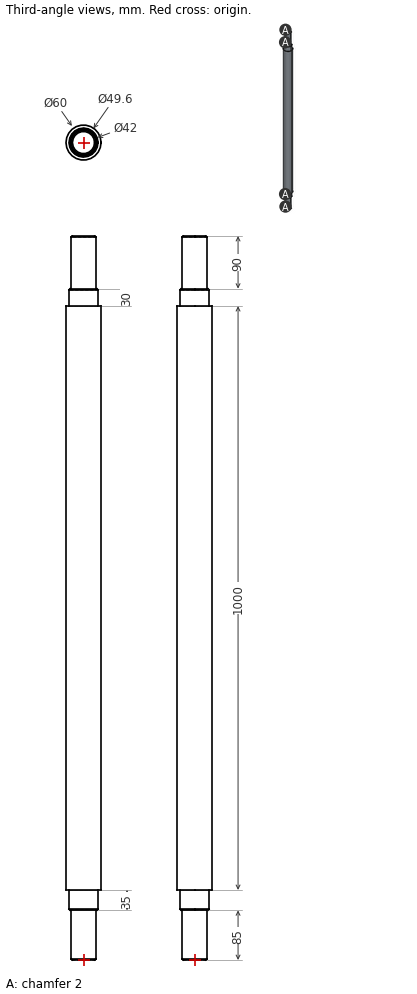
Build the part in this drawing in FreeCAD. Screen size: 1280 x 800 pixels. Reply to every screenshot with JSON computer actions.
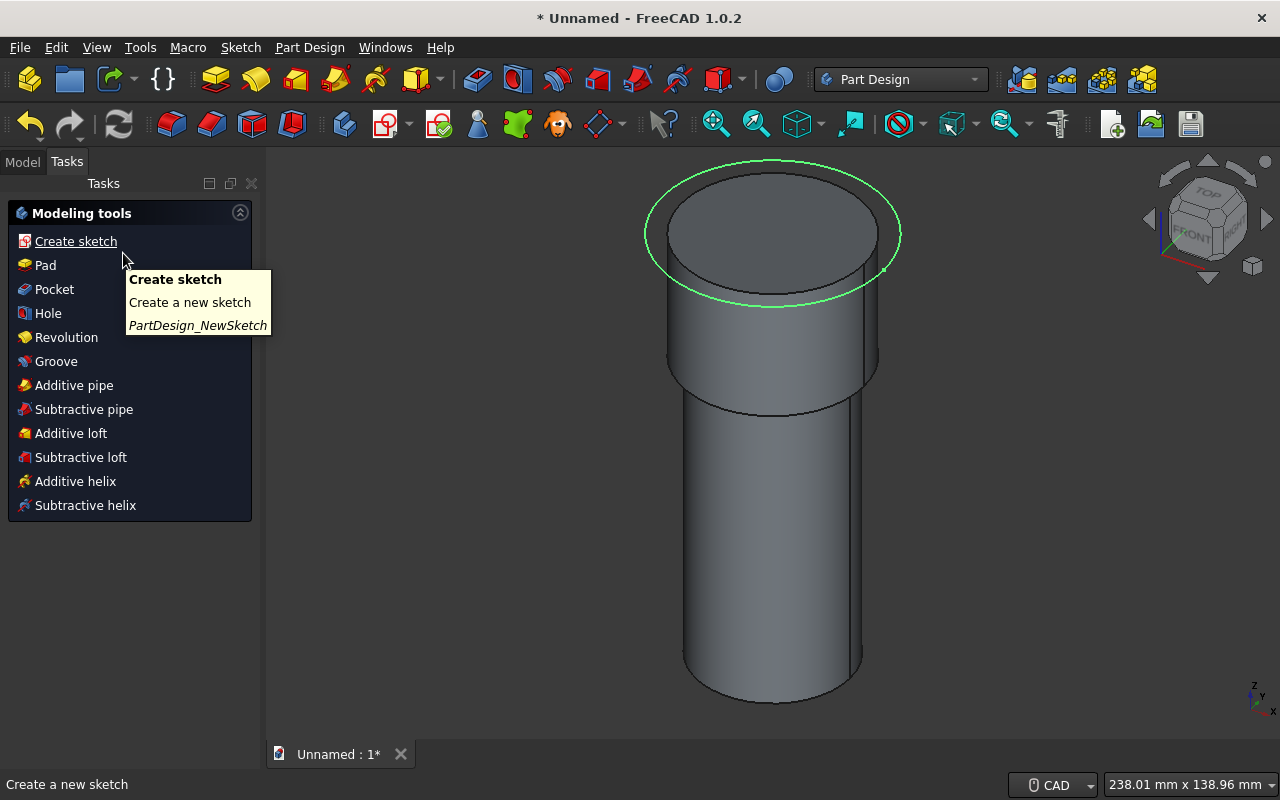
{"action": "left_click", "coordinate": [216, 80]}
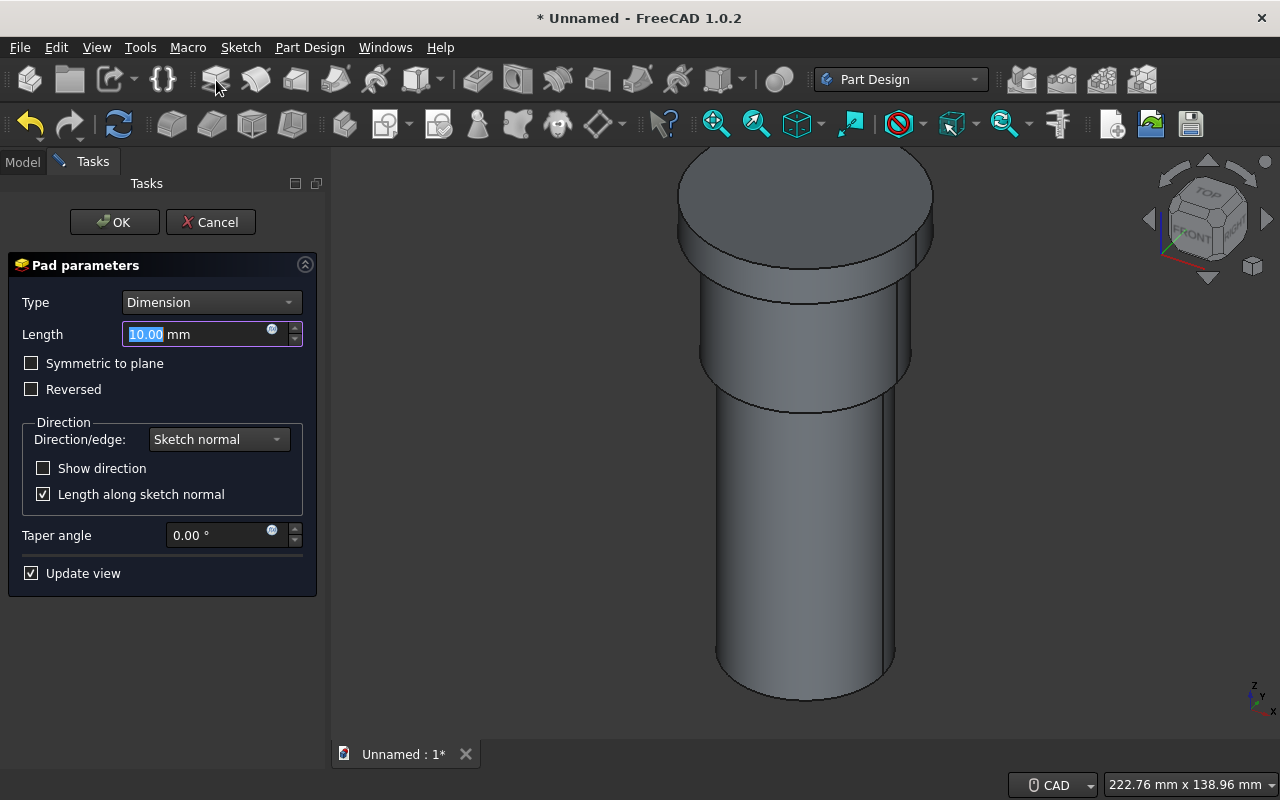
{"action": "type", "text": "1000"}
{"action": "key", "text": "Tab"}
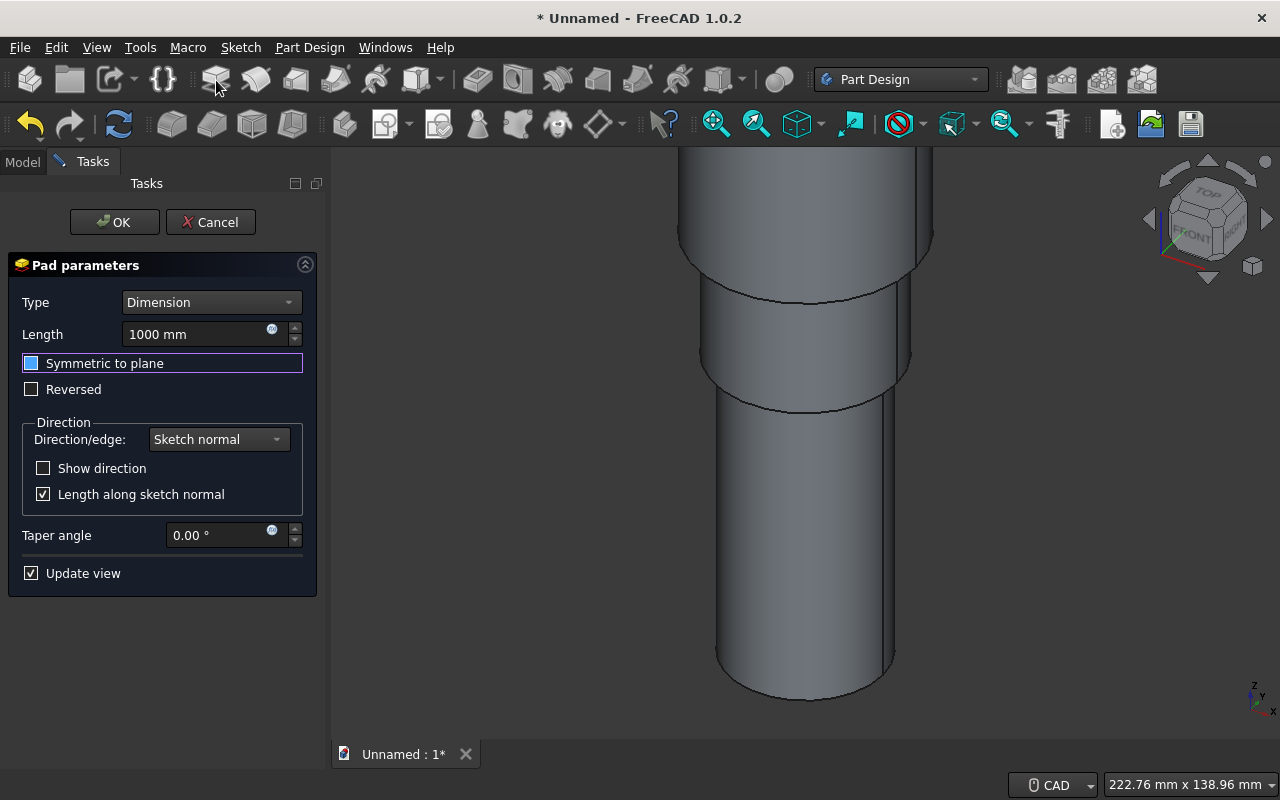
{"action": "left_click", "coordinate": [115, 222]}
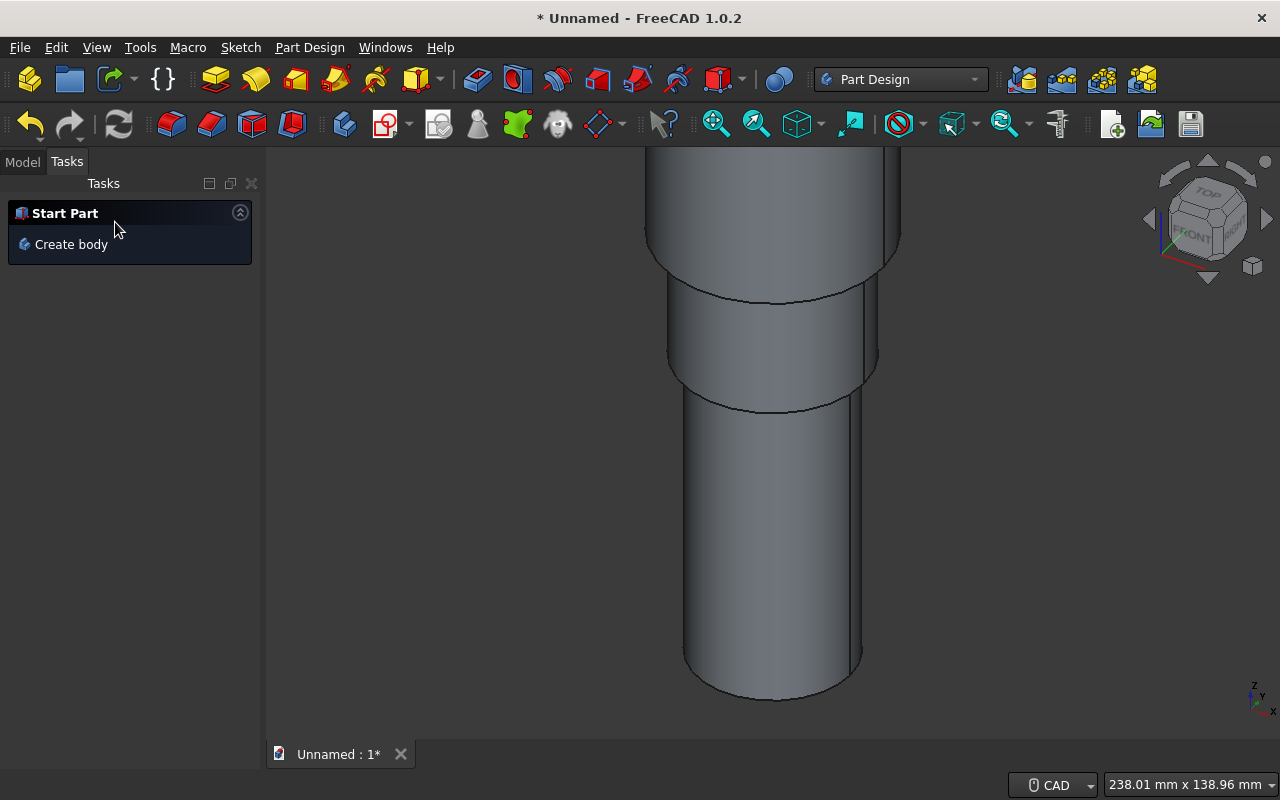
{"action": "key", "text": "v f"}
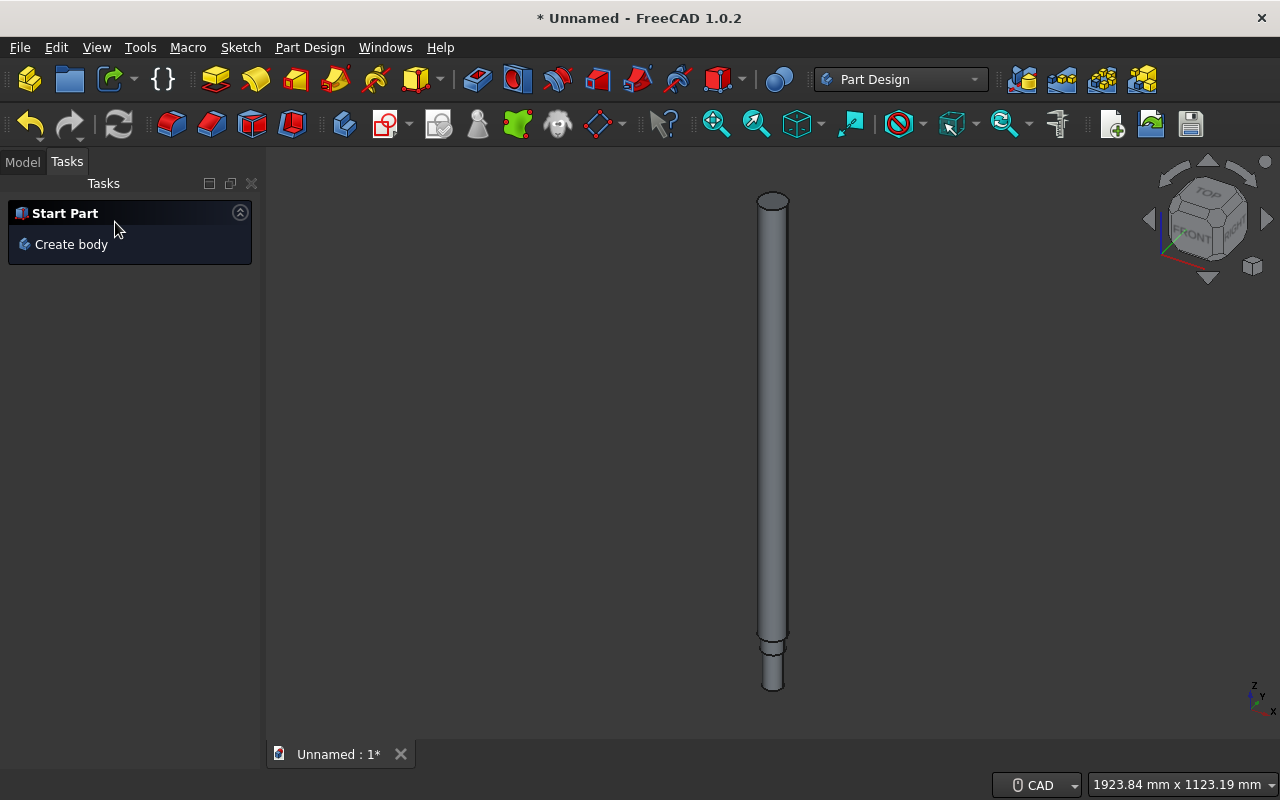
{"action": "left_click", "coordinate": [773, 200]}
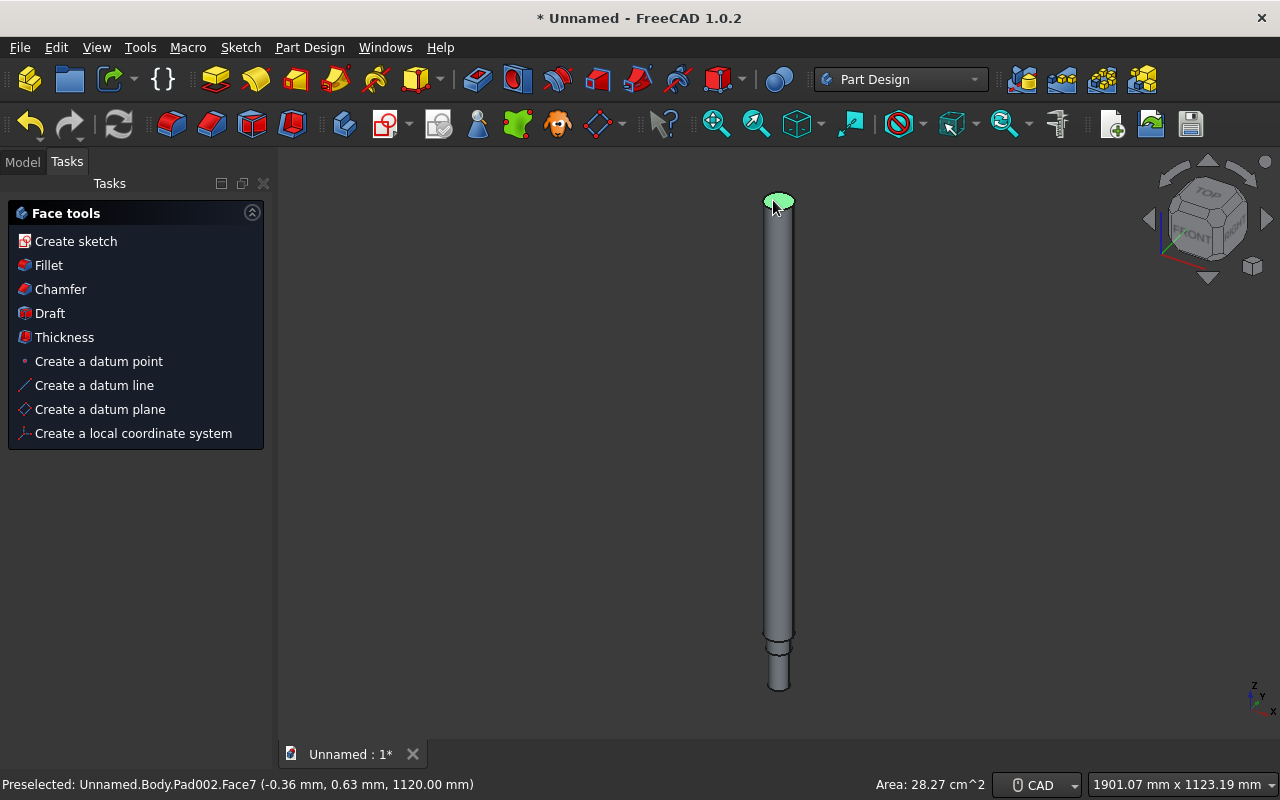
{"action": "left_click", "coordinate": [386, 124]}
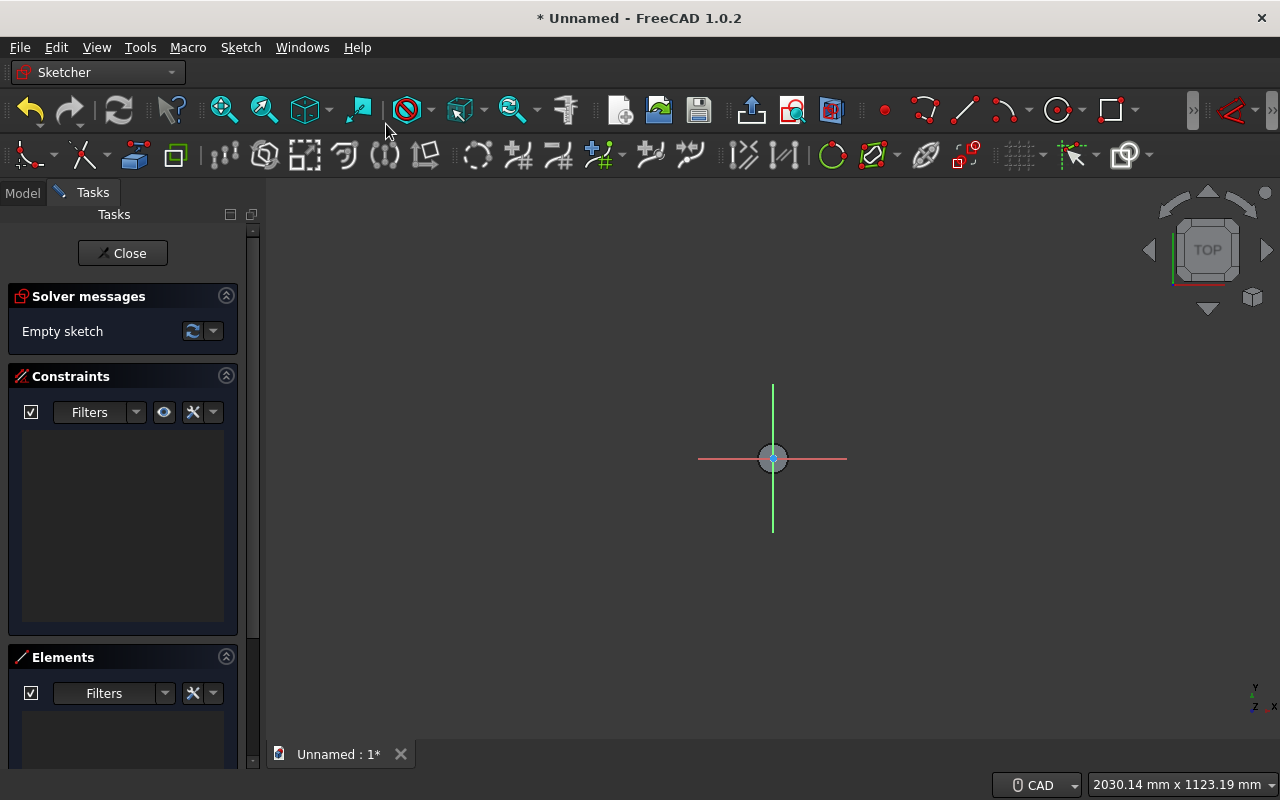
{"action": "scroll", "coordinate": [778, 458], "scroll_direction": "up", "scroll_amount": 13}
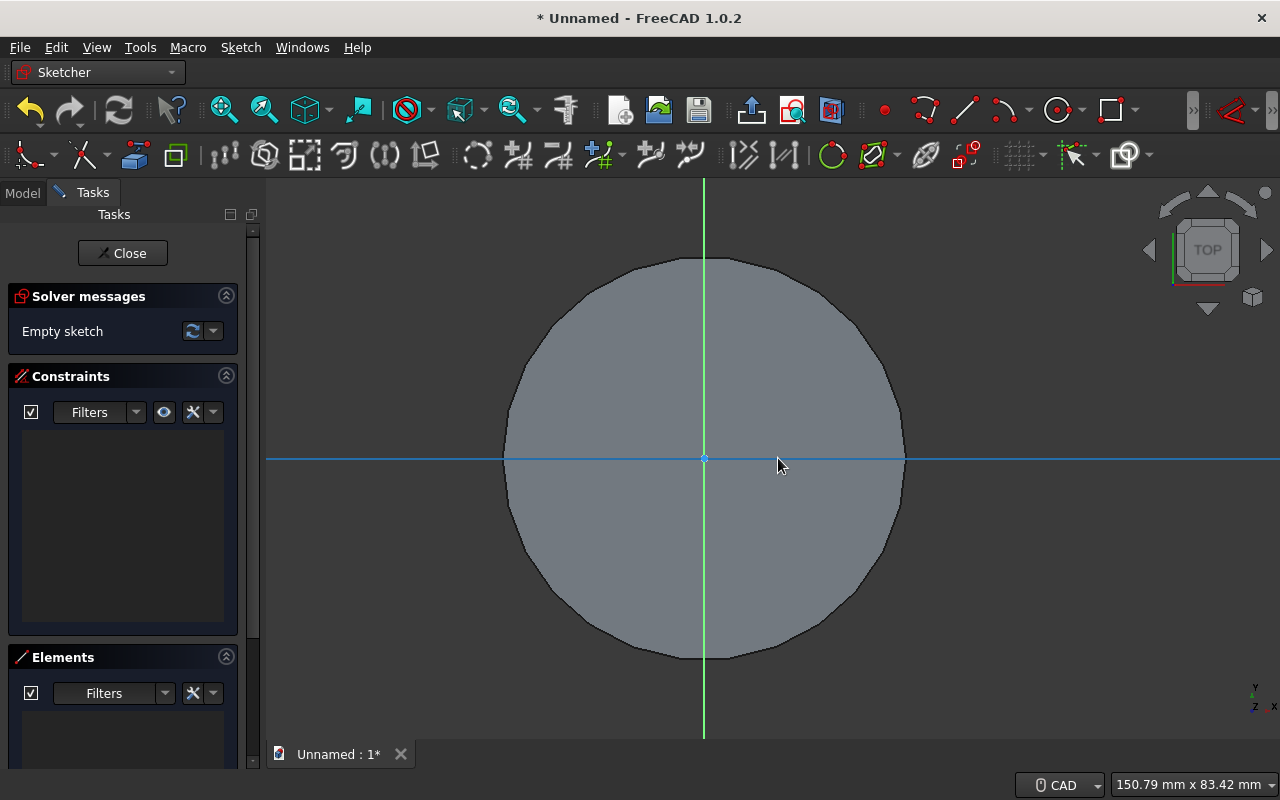
{"action": "key", "text": "g c"}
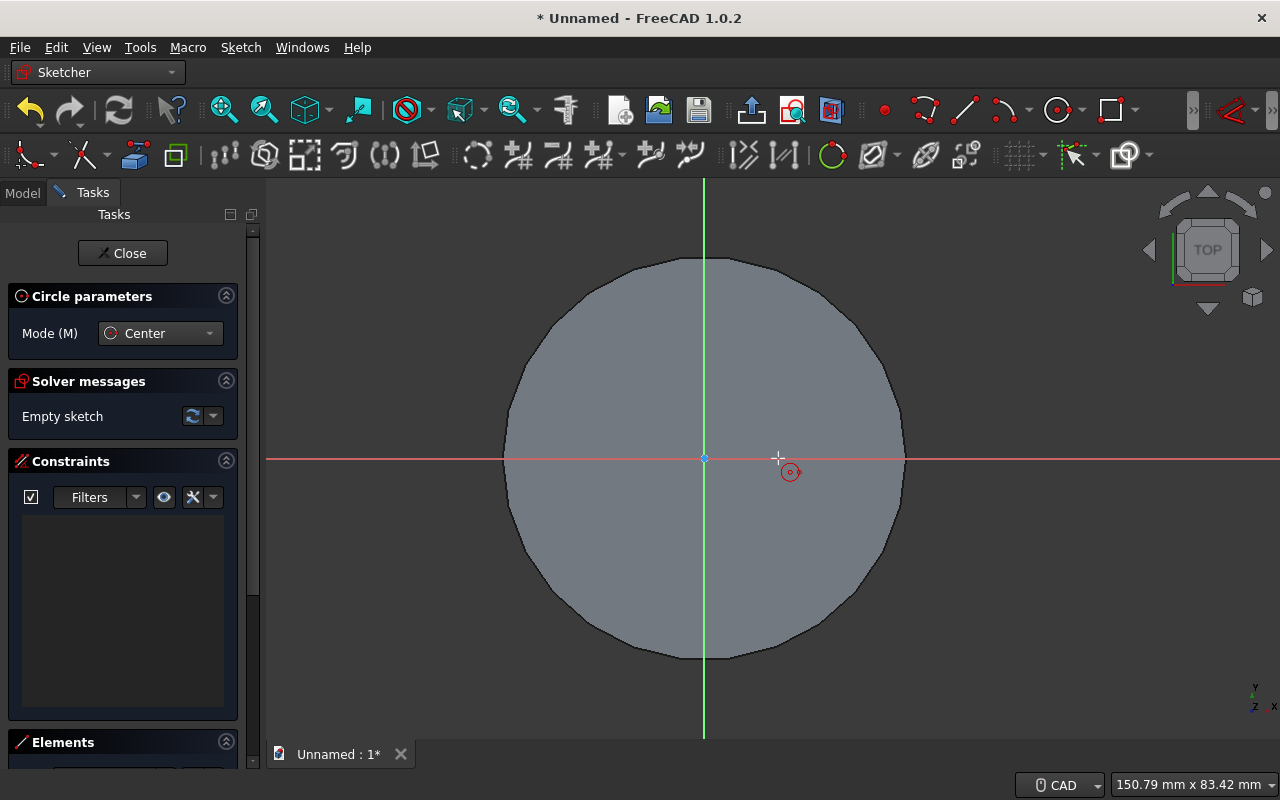
{"action": "left_click", "coordinate": [704, 458]}
{"action": "mouse_move", "coordinate": [822, 341]}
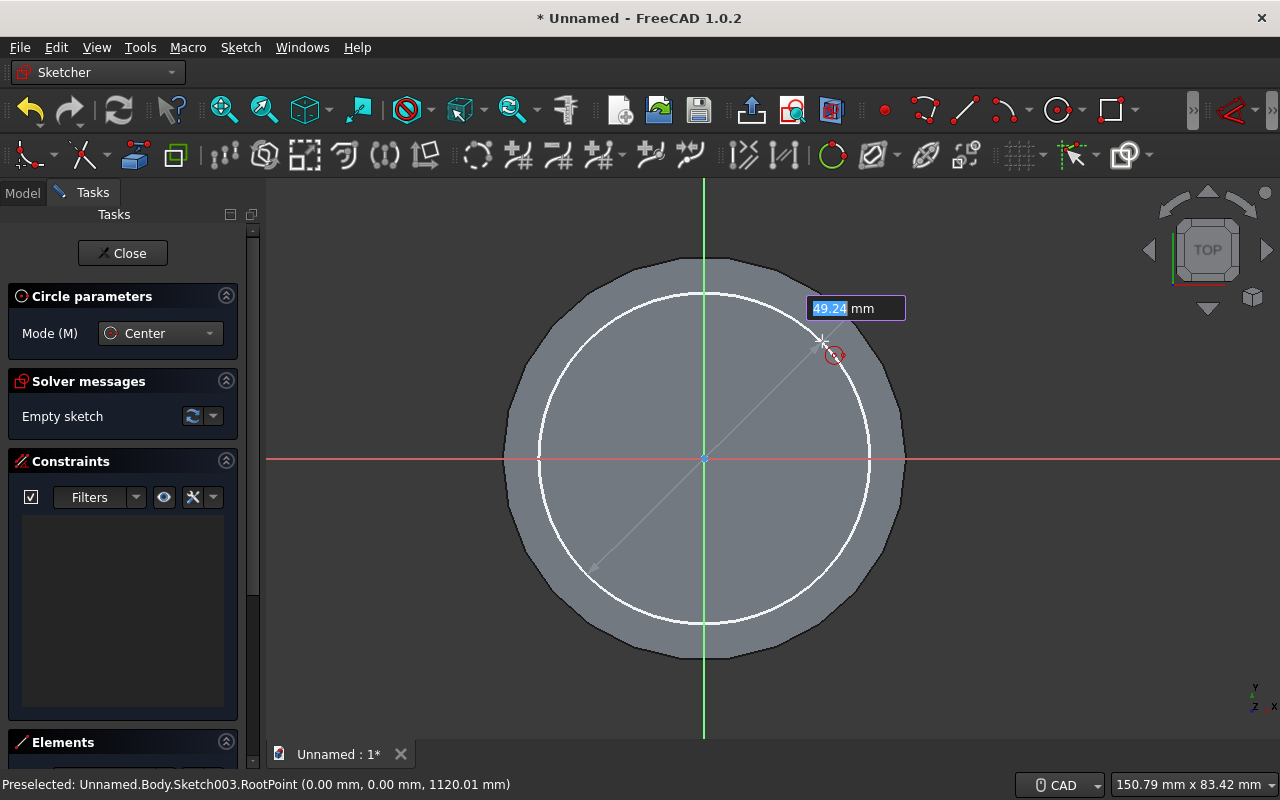
{"action": "type", "text": "49.6"}
{"action": "key", "text": "Return"}
{"action": "key", "text": "Escape"}